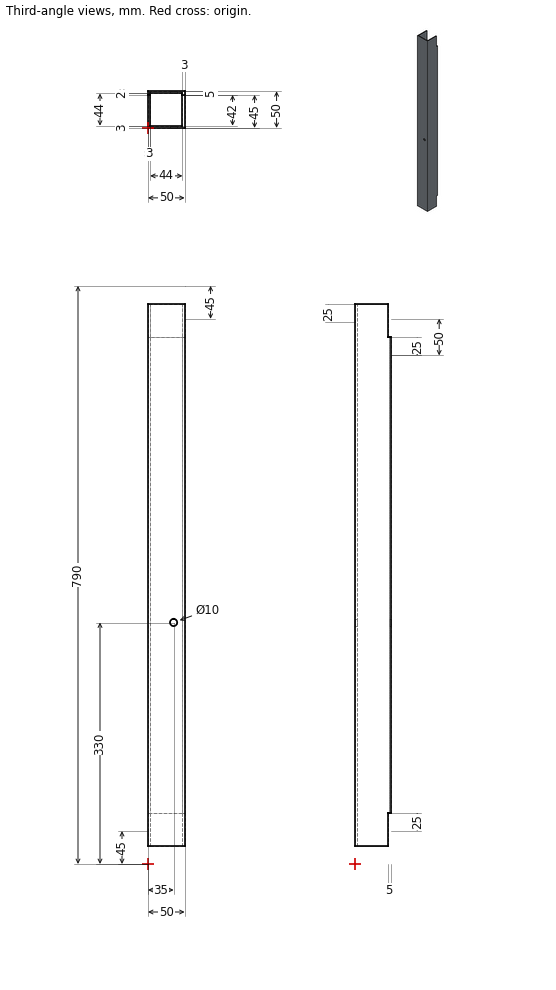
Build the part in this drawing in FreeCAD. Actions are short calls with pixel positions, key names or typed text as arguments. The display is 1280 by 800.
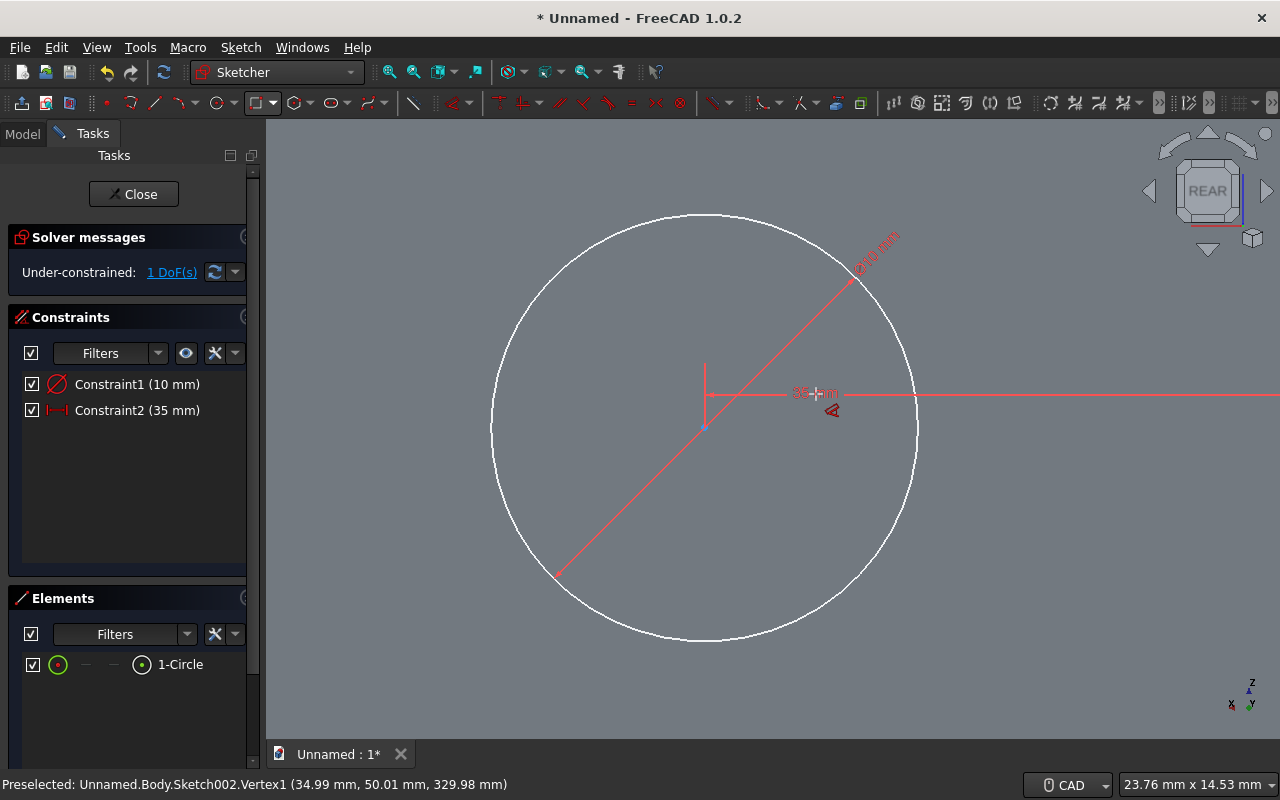
click(705, 428)
click(671, 569)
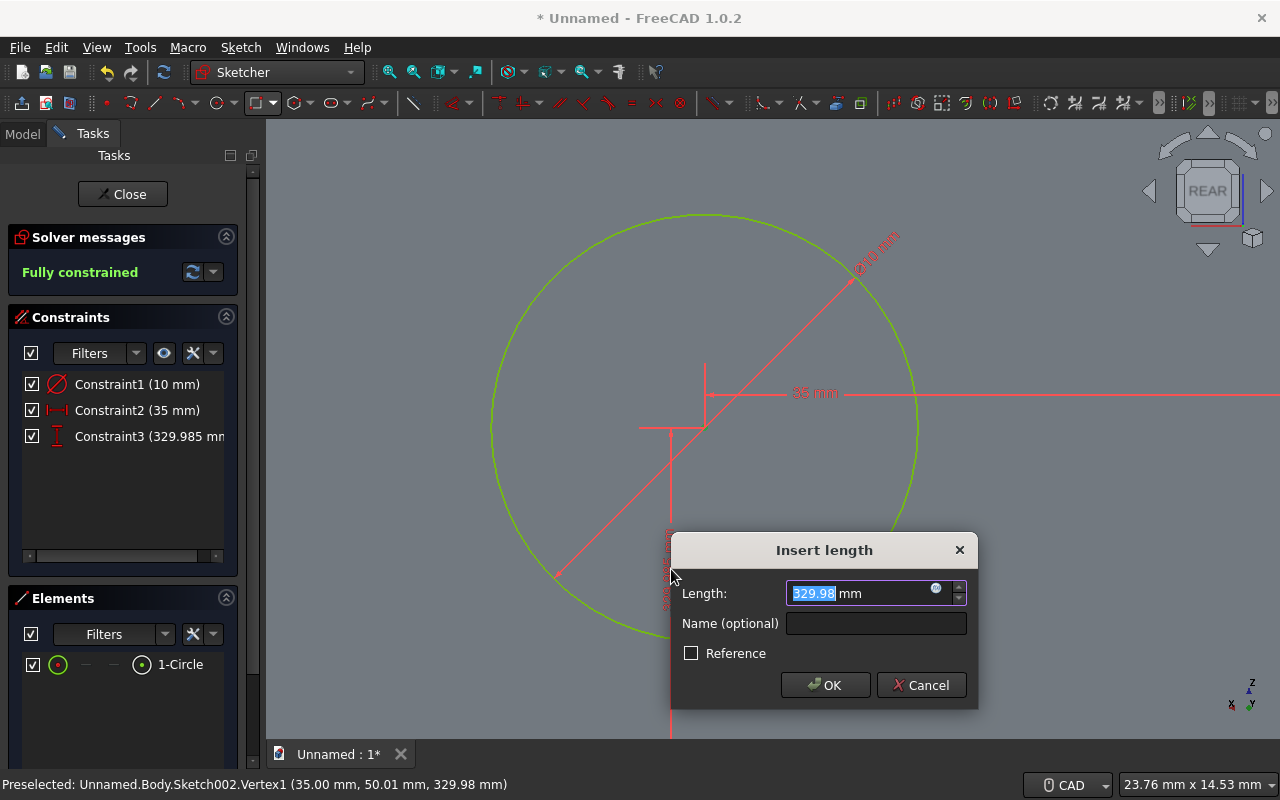
text(330)
key(Return)
key(Escape)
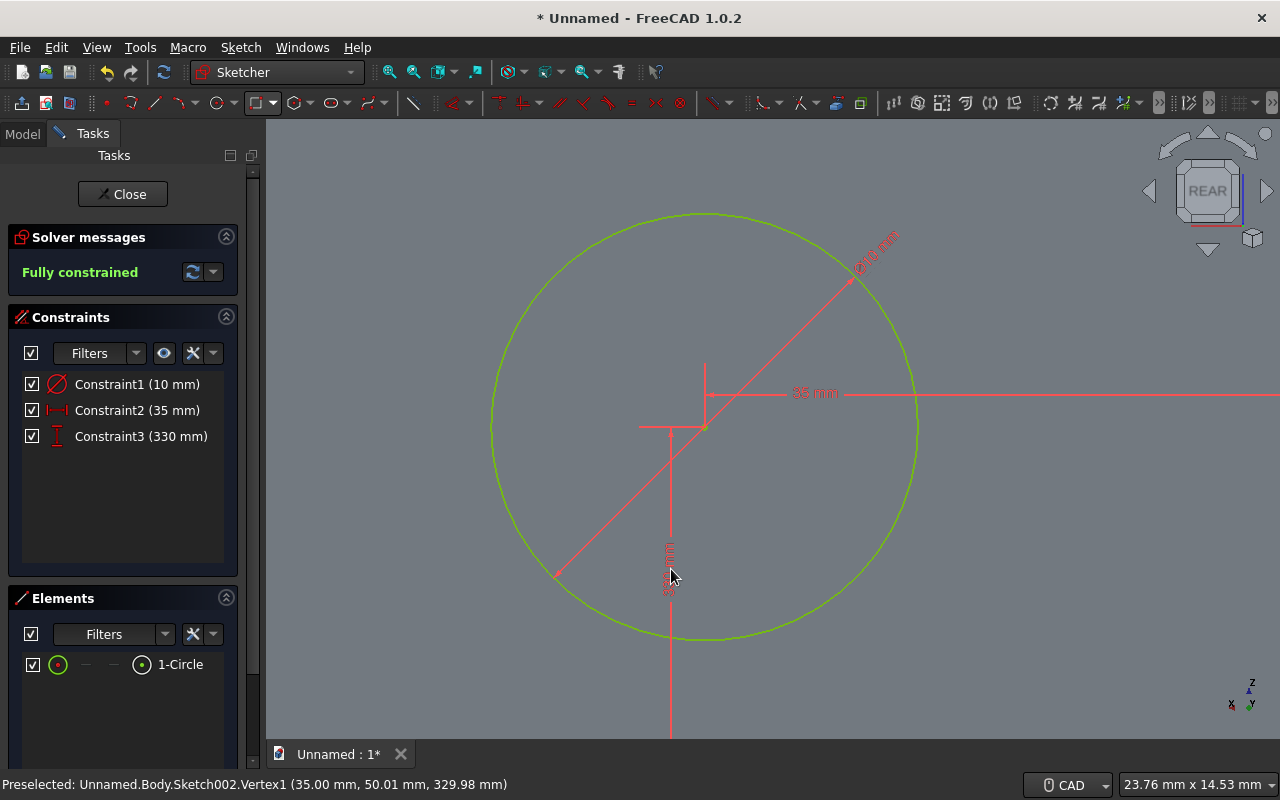
click(123, 194)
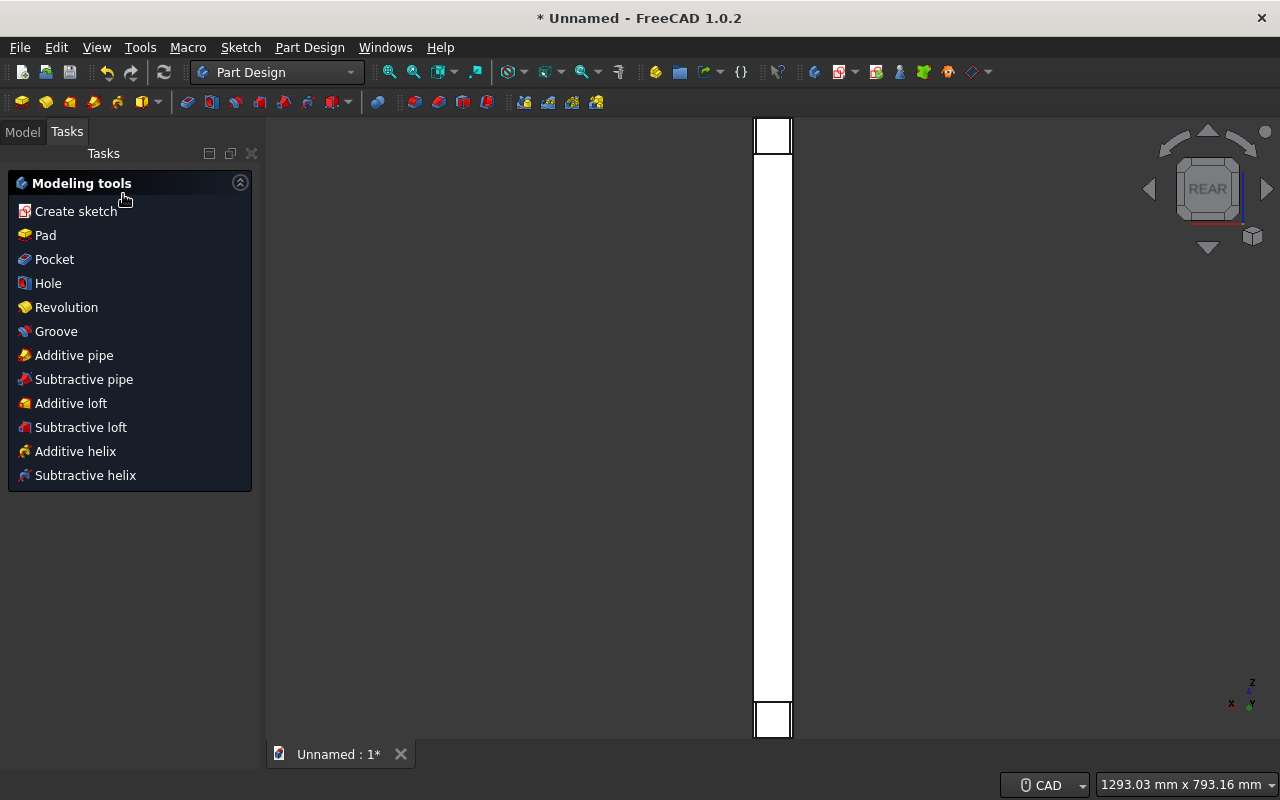
click(188, 102)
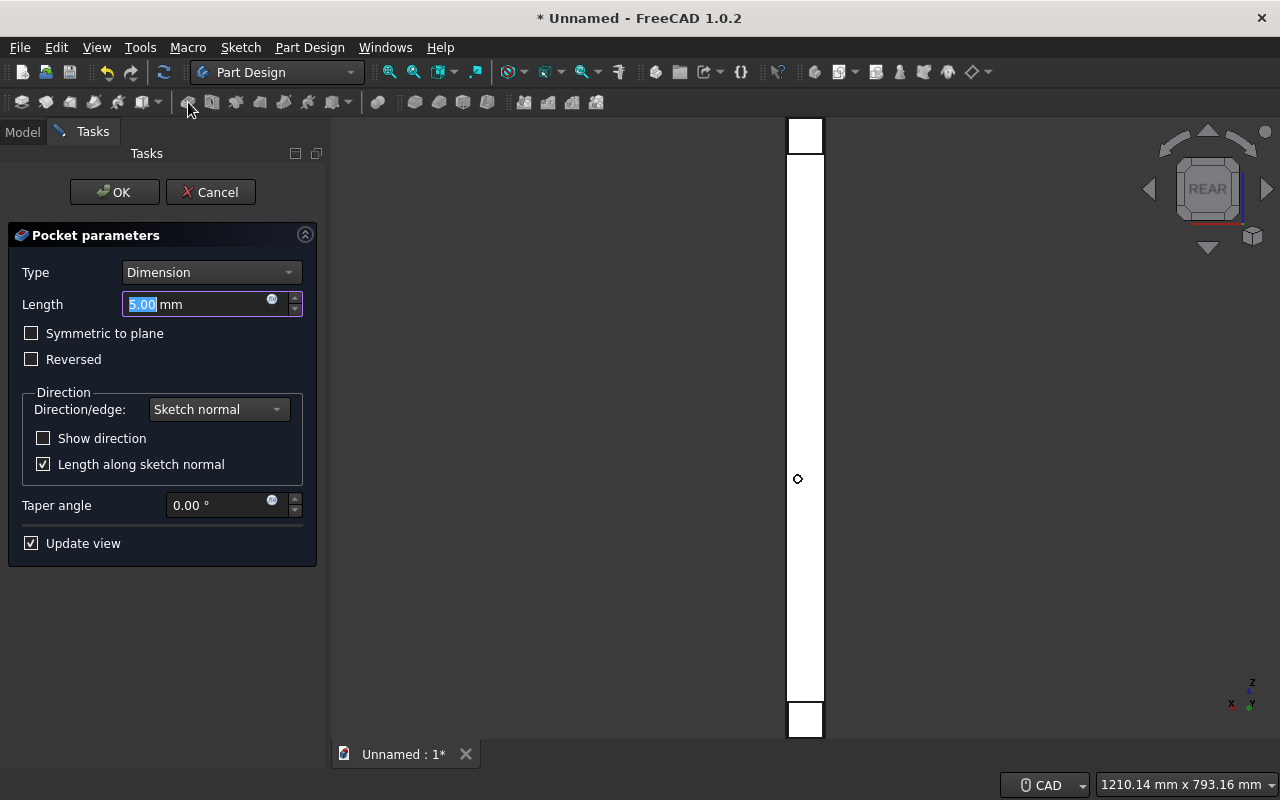
text(5)
key(Tab)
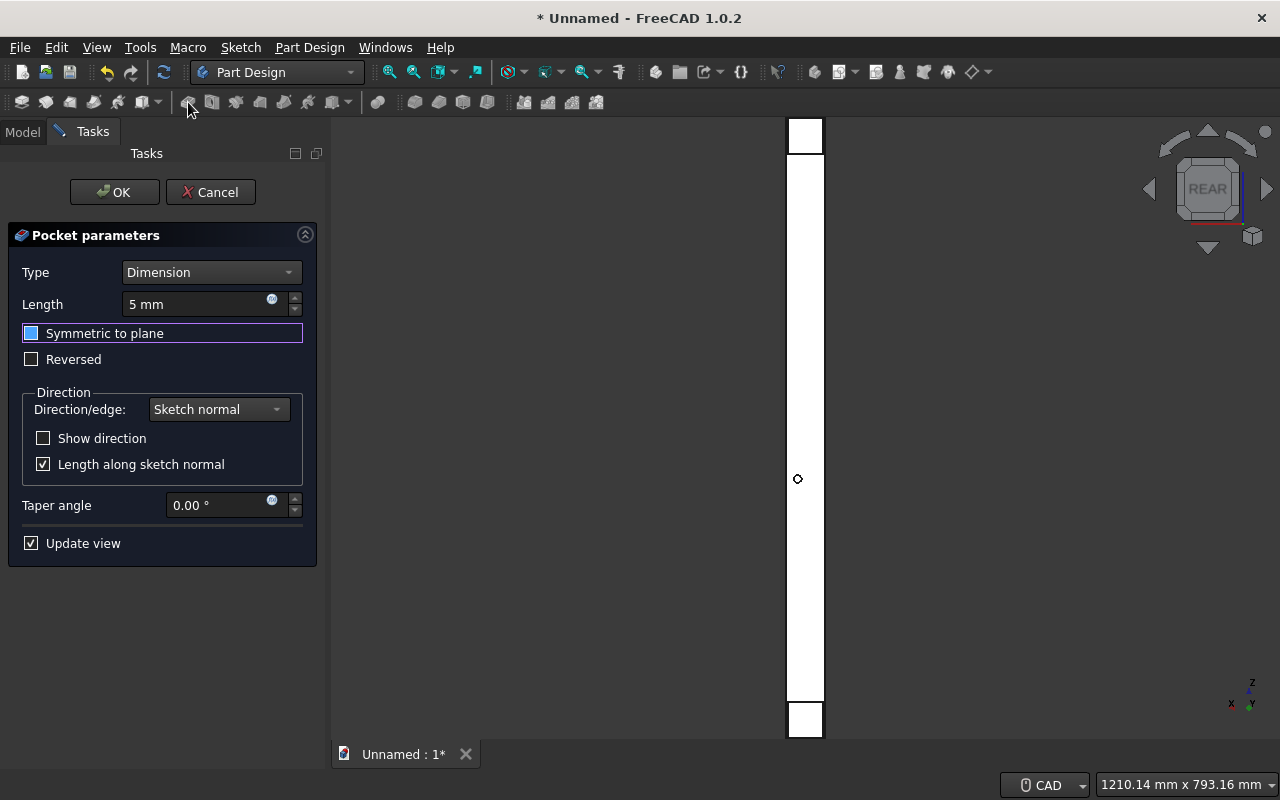
click(115, 192)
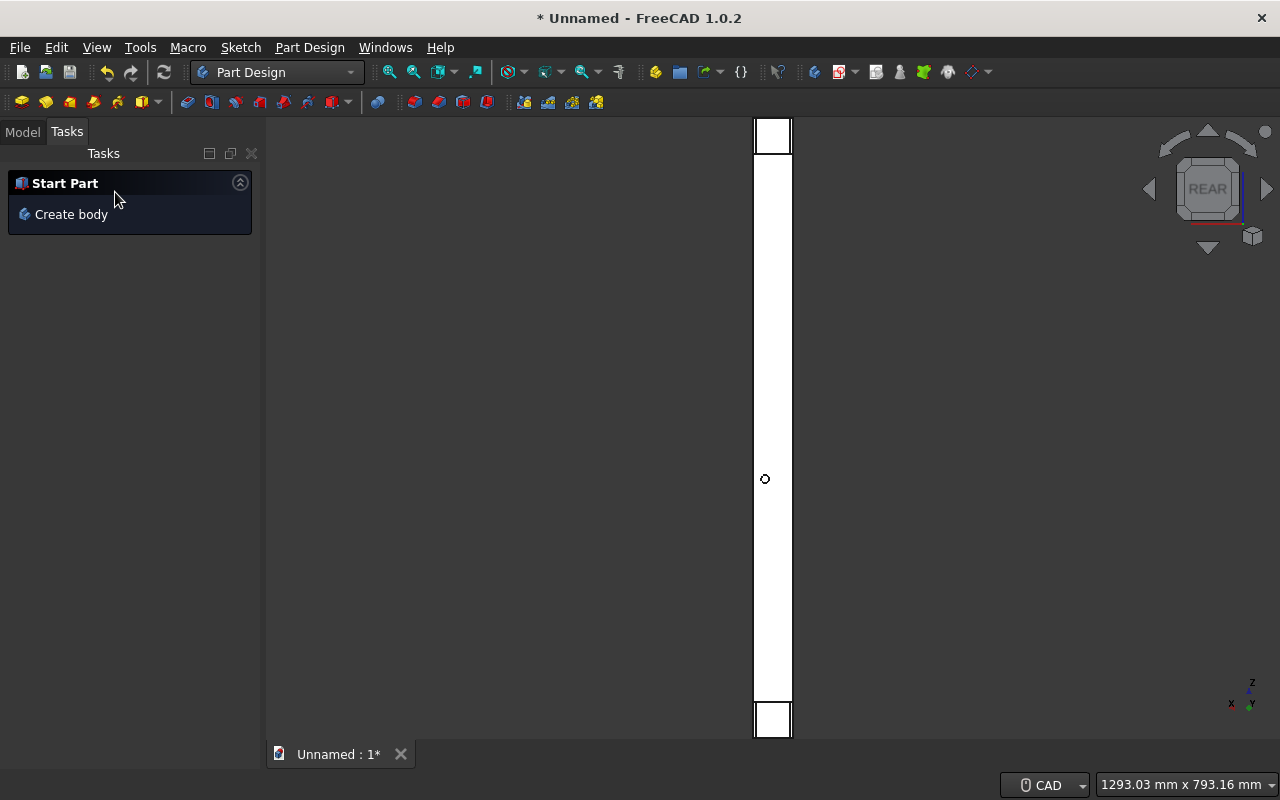
key(0)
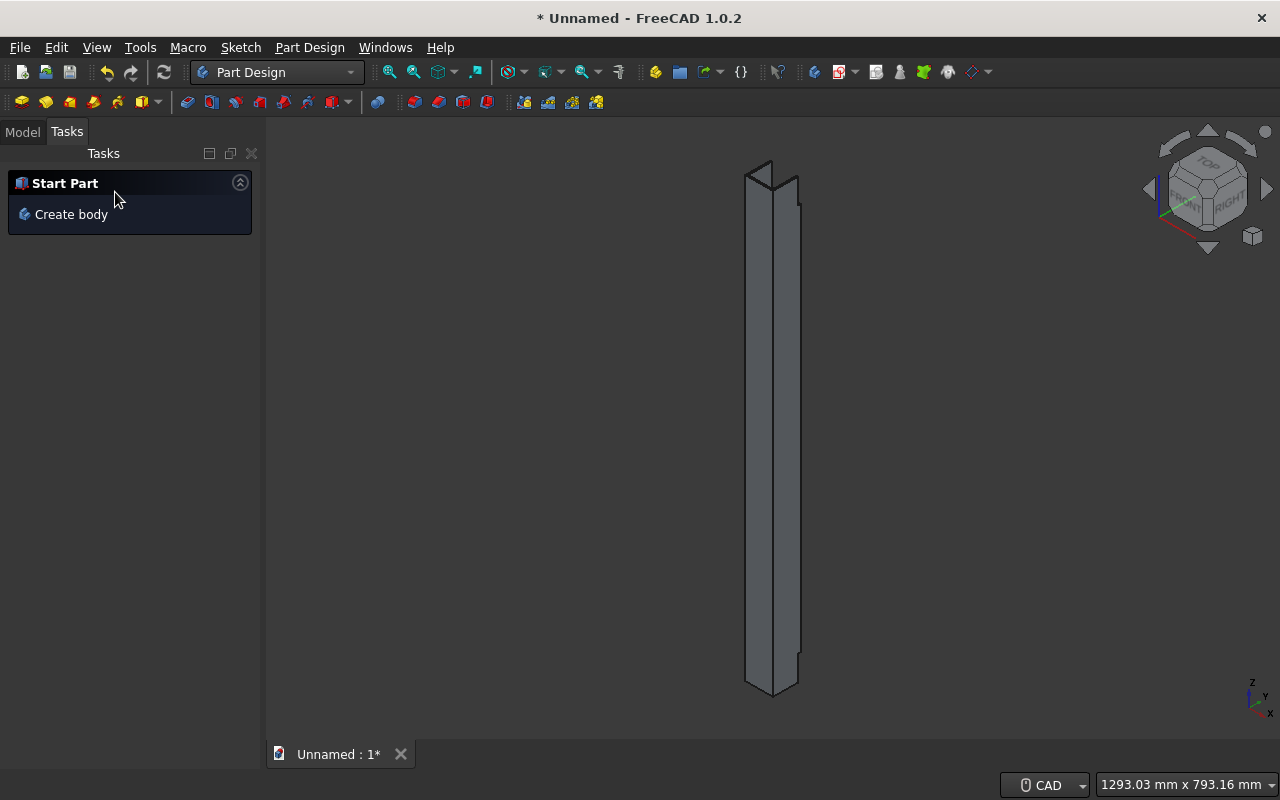
scroll(781, 185, up, 14)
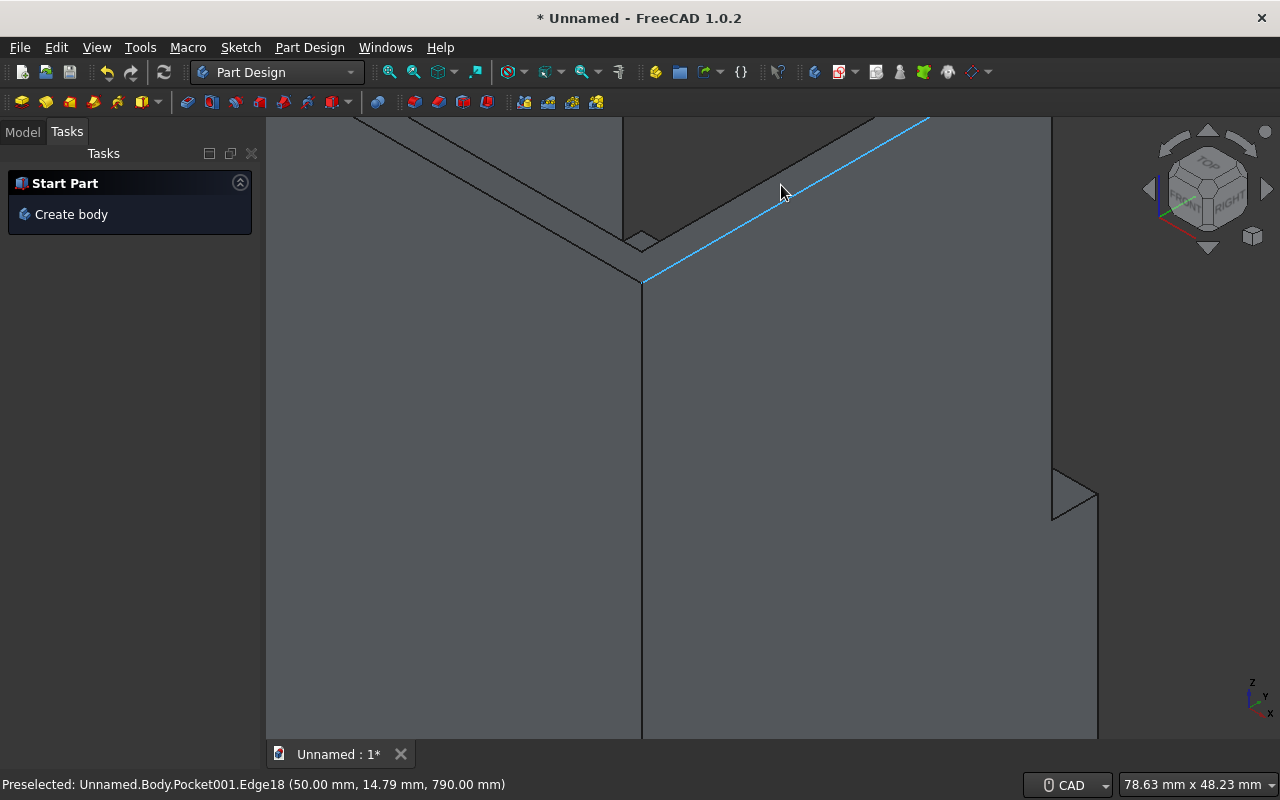
click(778, 193)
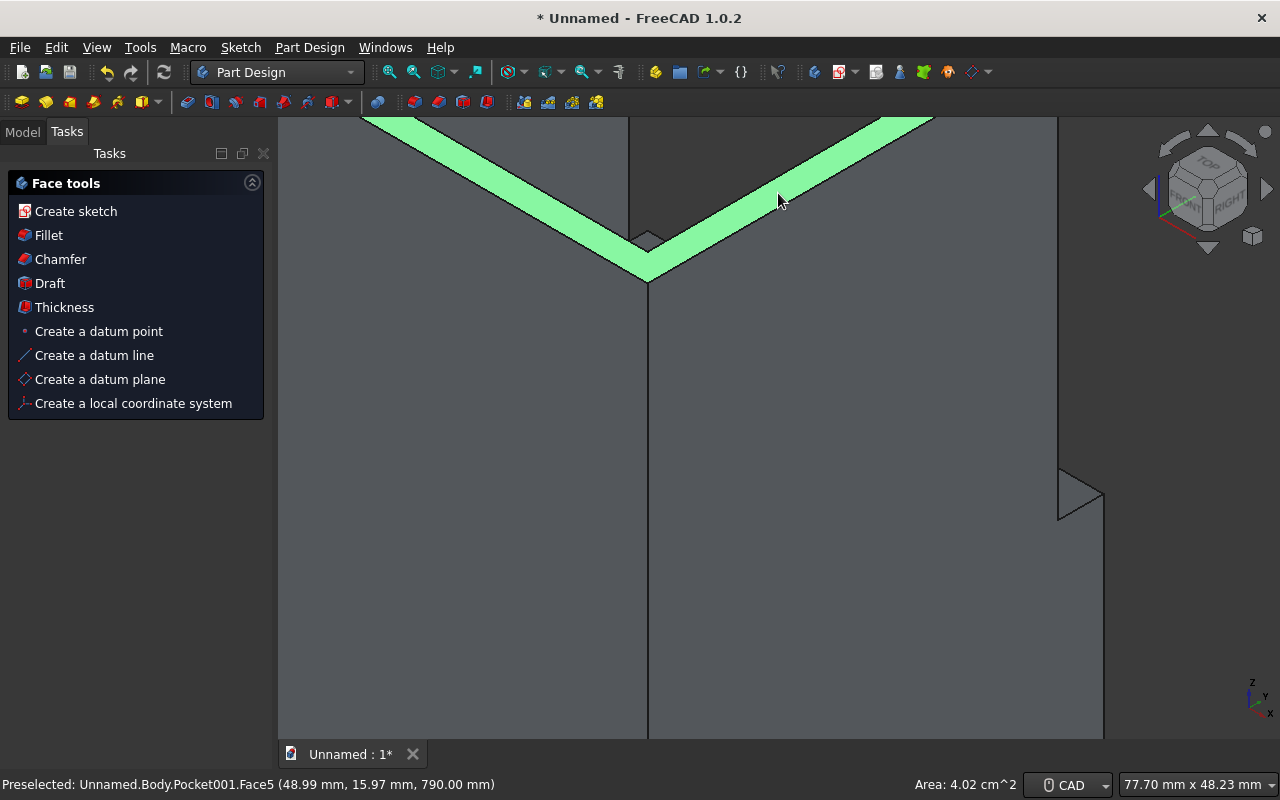
click(840, 72)